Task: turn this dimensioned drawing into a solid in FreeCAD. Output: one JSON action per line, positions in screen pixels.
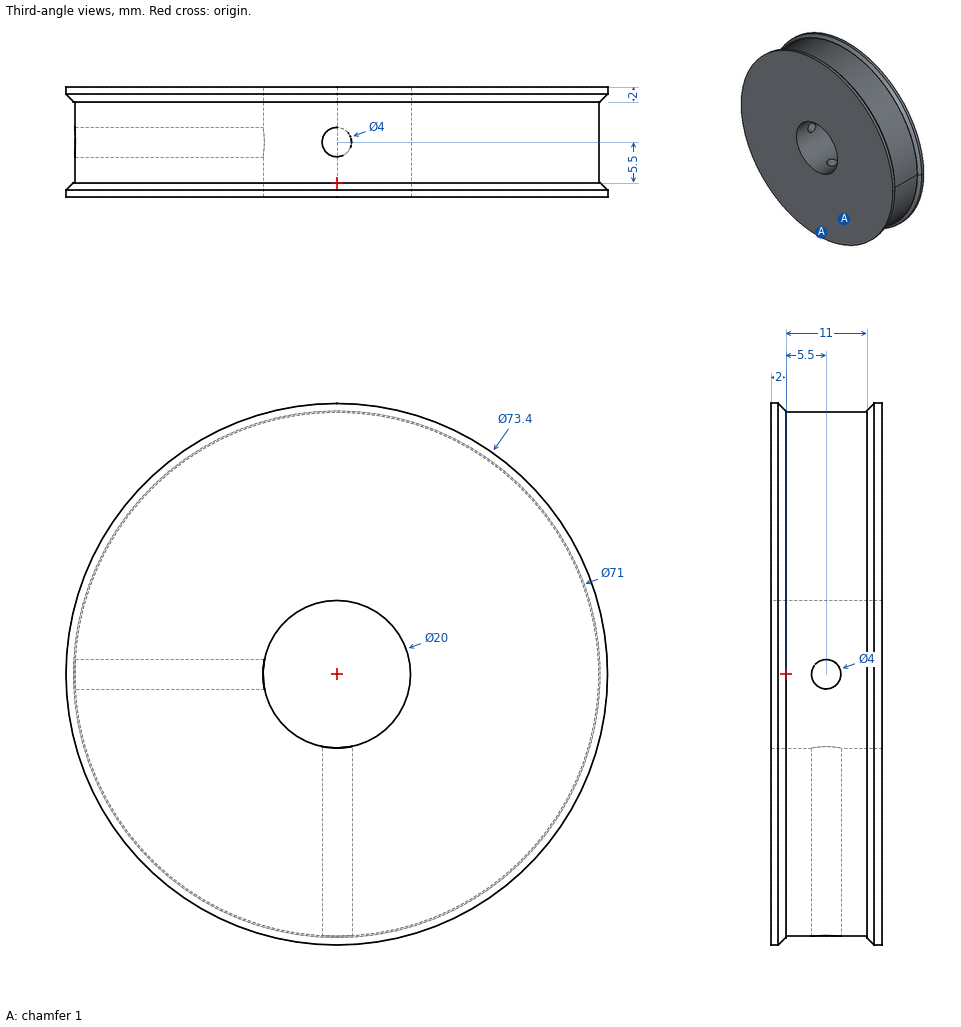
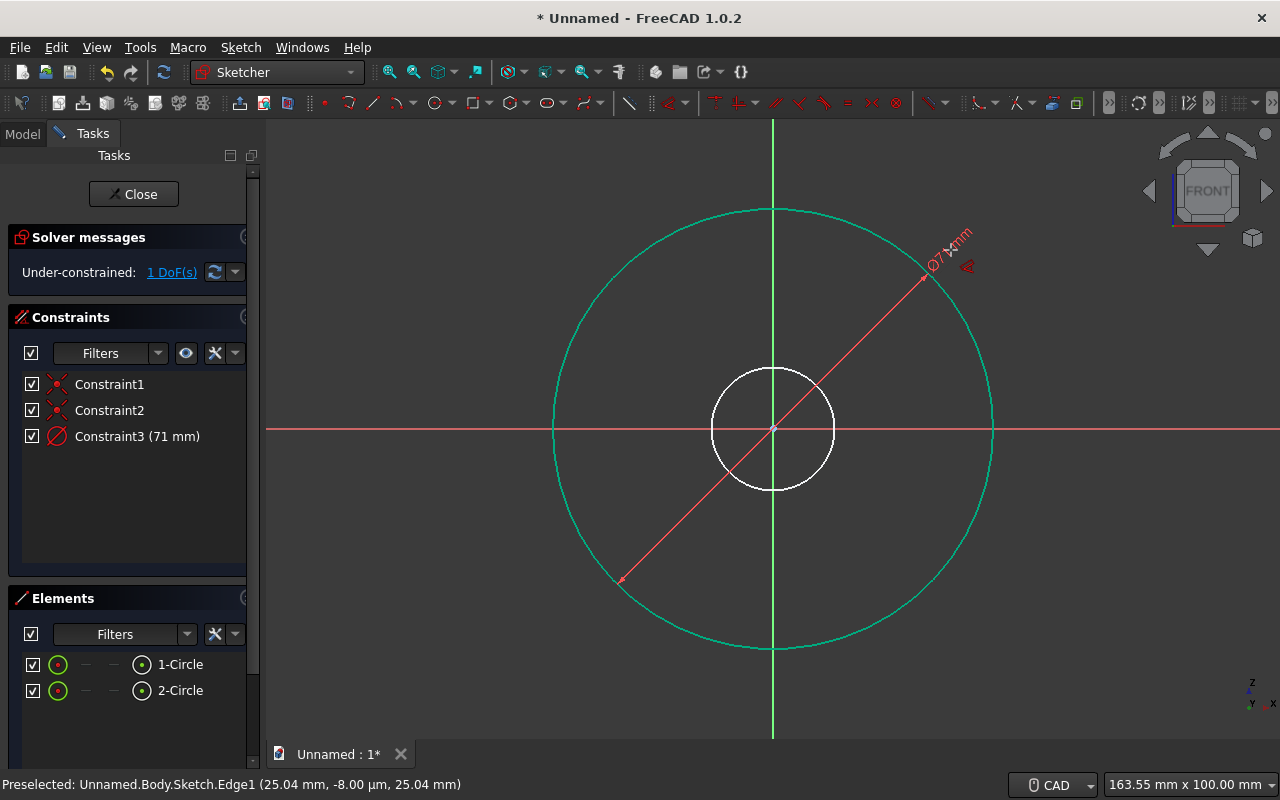
{"action": "left_click", "coordinate": [816, 385]}
{"action": "left_click", "coordinate": [838, 362]}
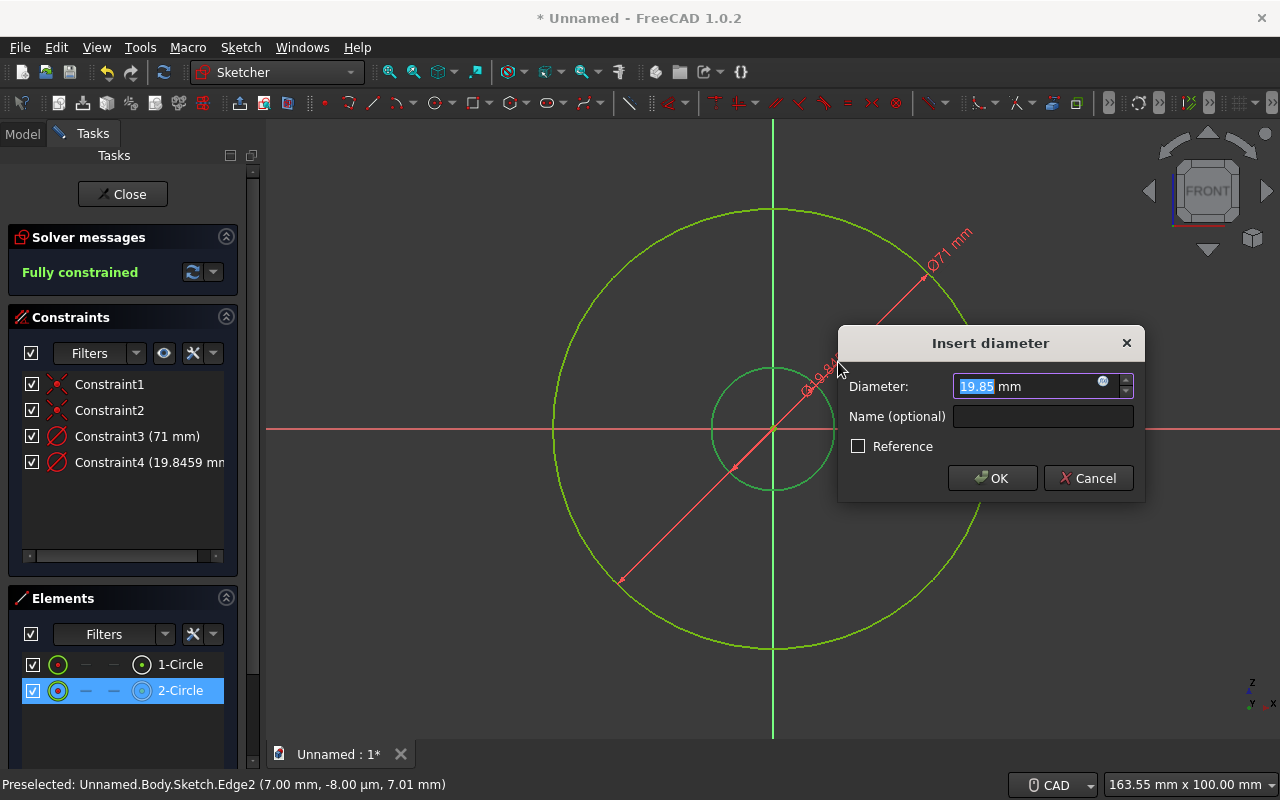
{"action": "type", "text": "20"}
{"action": "key", "text": "Return"}
{"action": "key", "text": "Escape"}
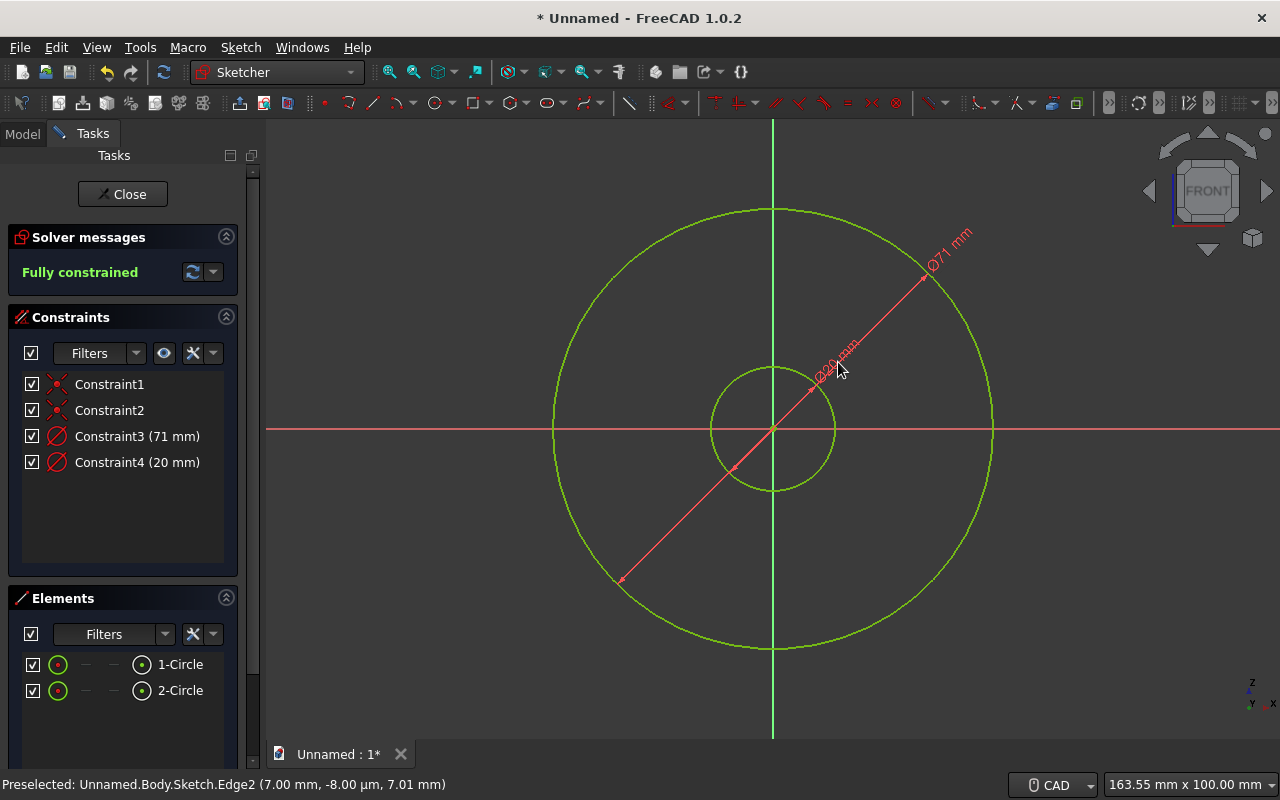
{"action": "left_click", "coordinate": [123, 194]}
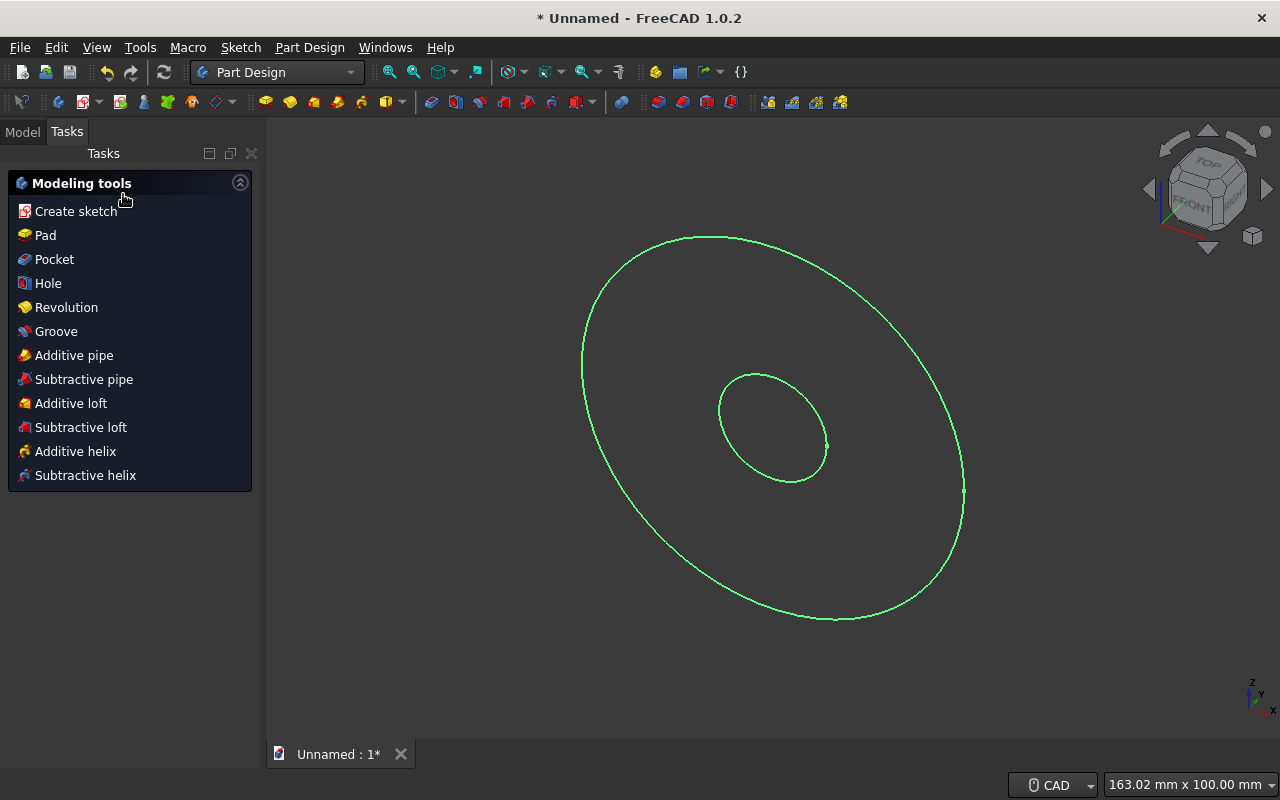
{"action": "left_click", "coordinate": [266, 102]}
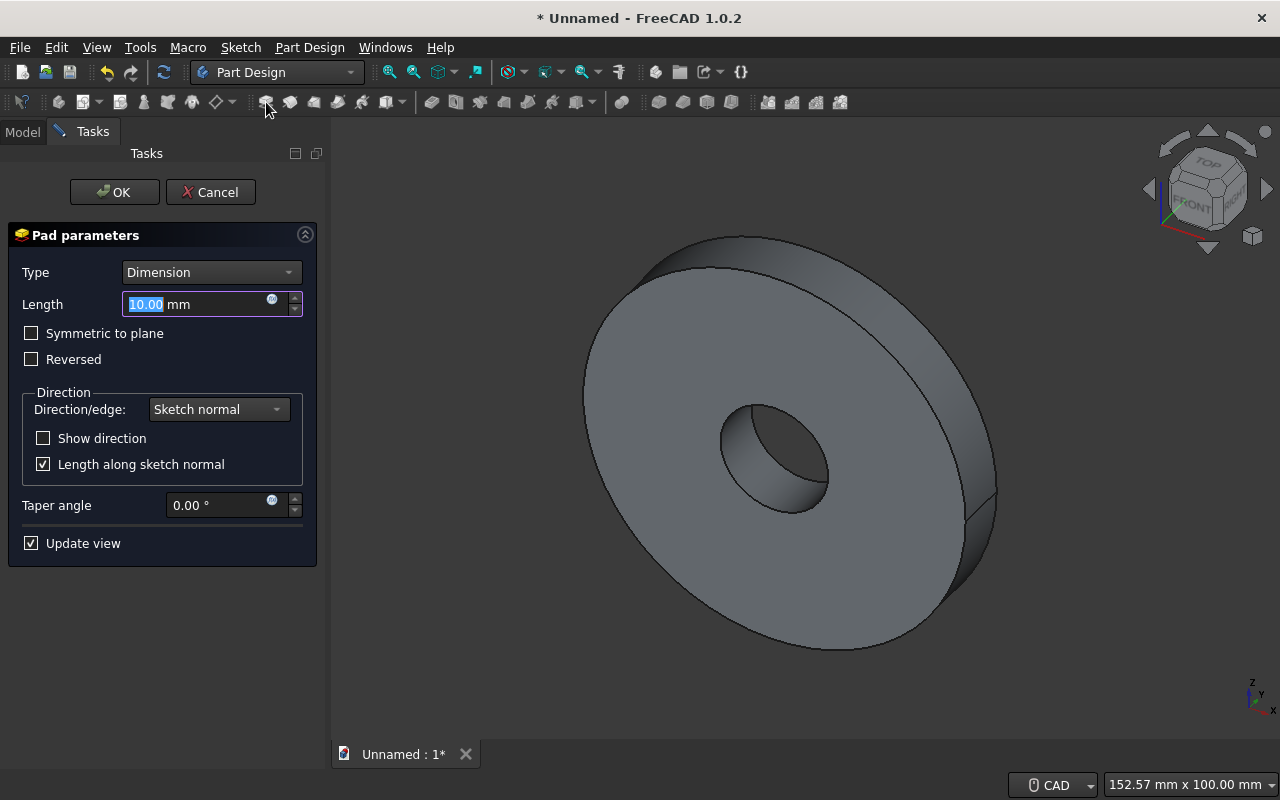
{"action": "type", "text": "11"}
{"action": "key", "text": "Tab"}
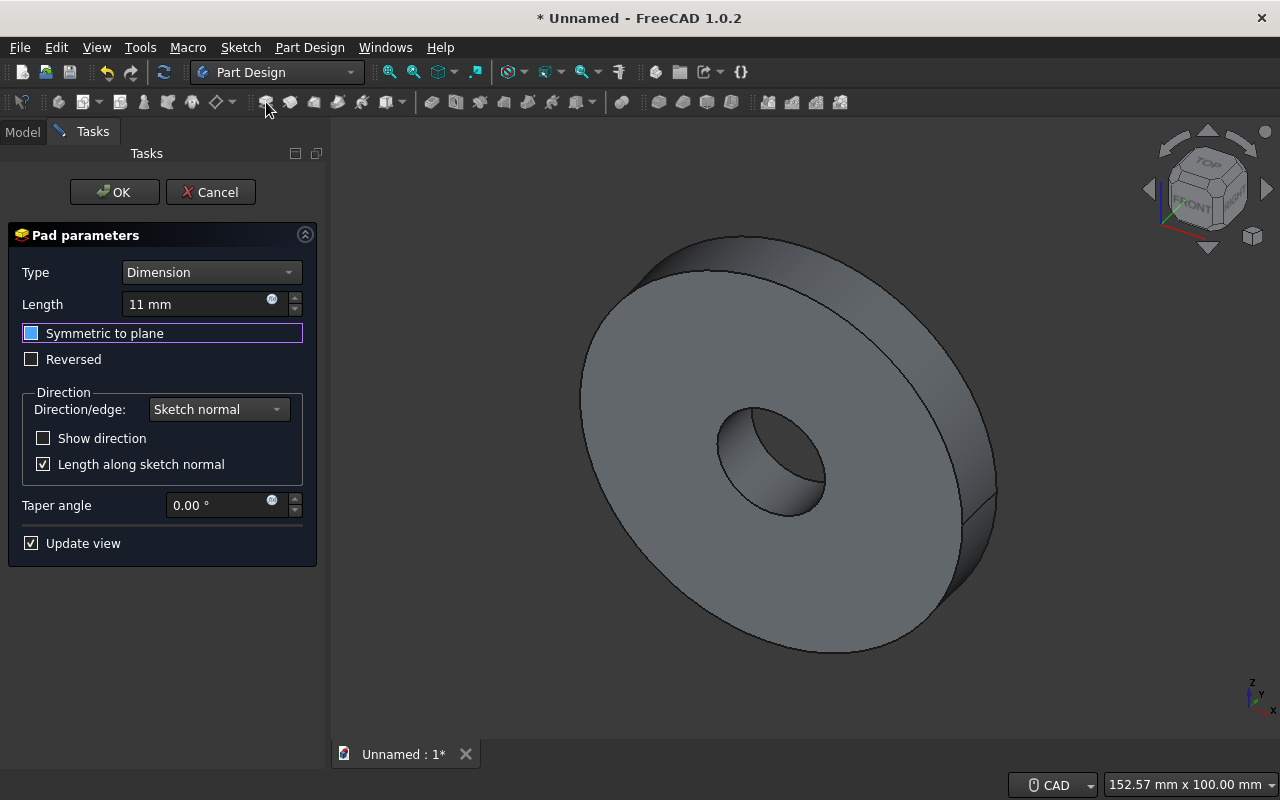
{"action": "left_click", "coordinate": [30, 359]}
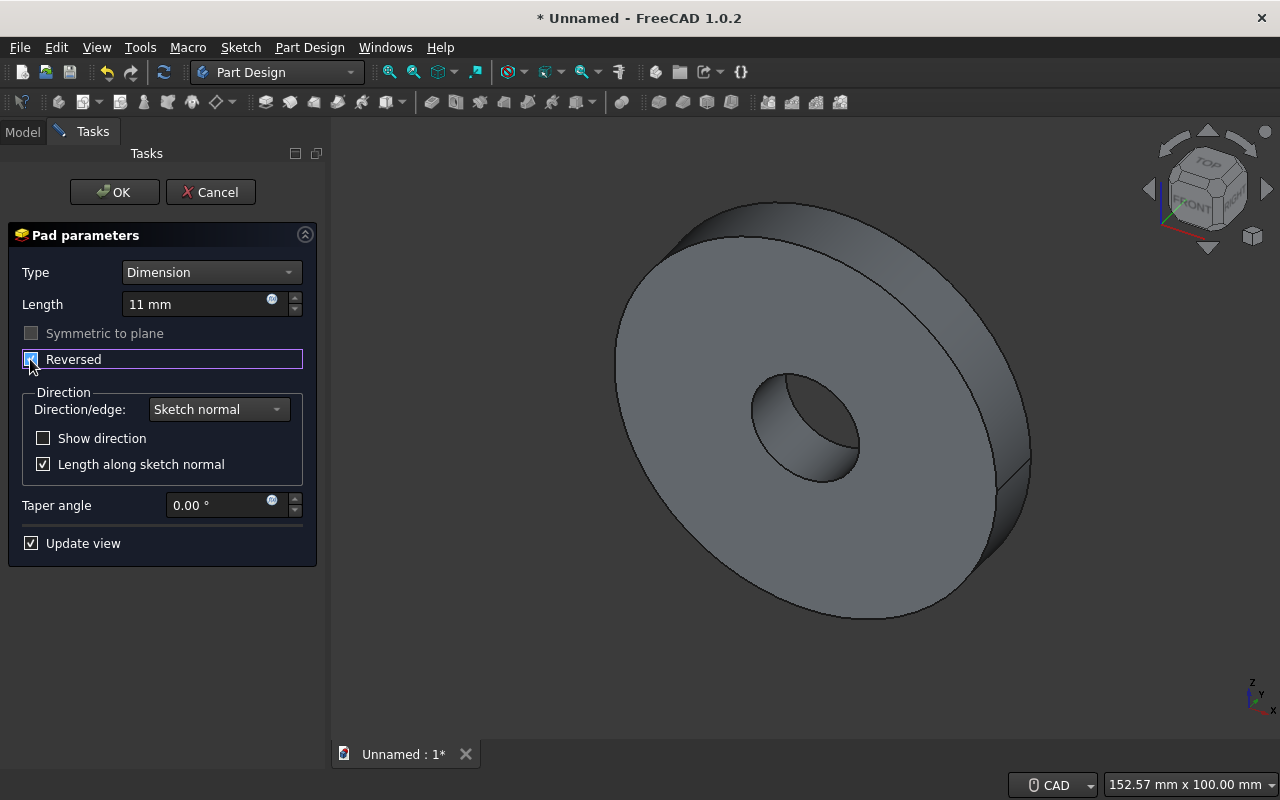
{"action": "left_click", "coordinate": [115, 192]}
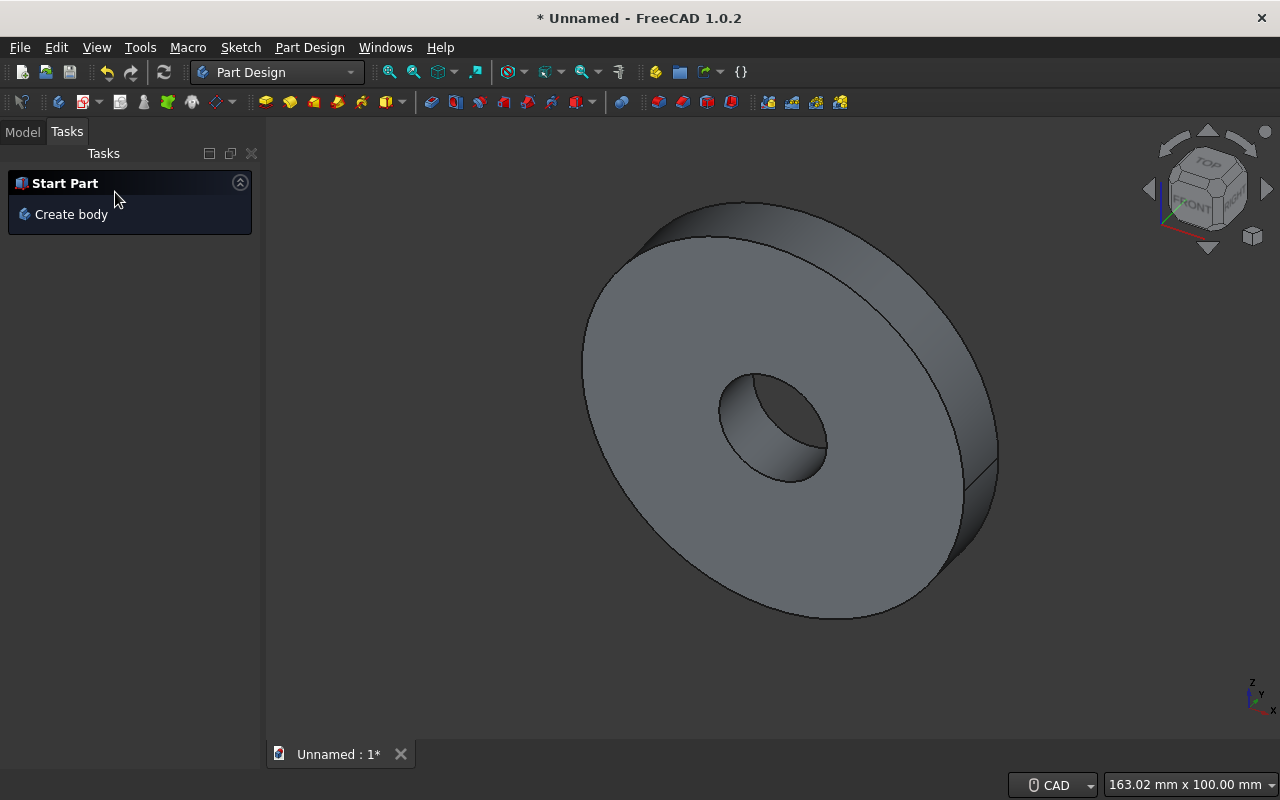
{"action": "key", "text": "4"}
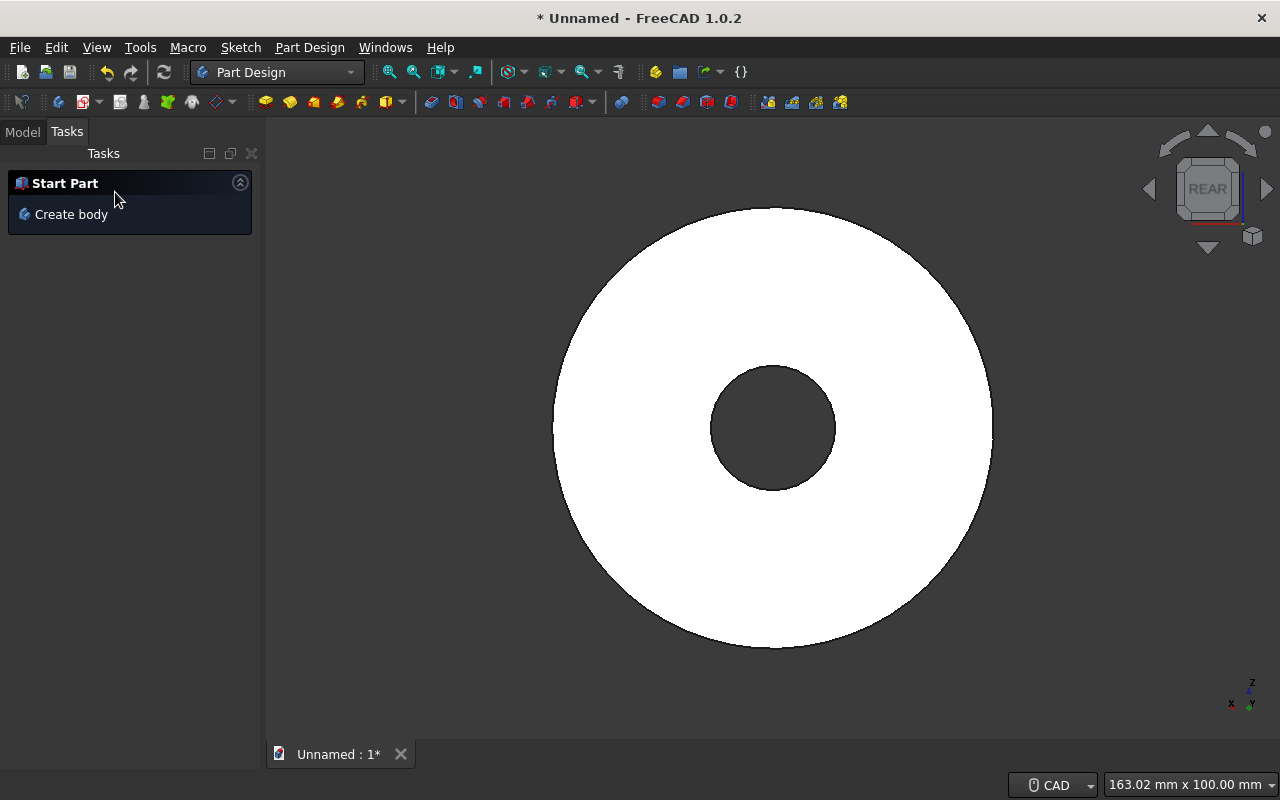
{"action": "left_click", "coordinate": [647, 364]}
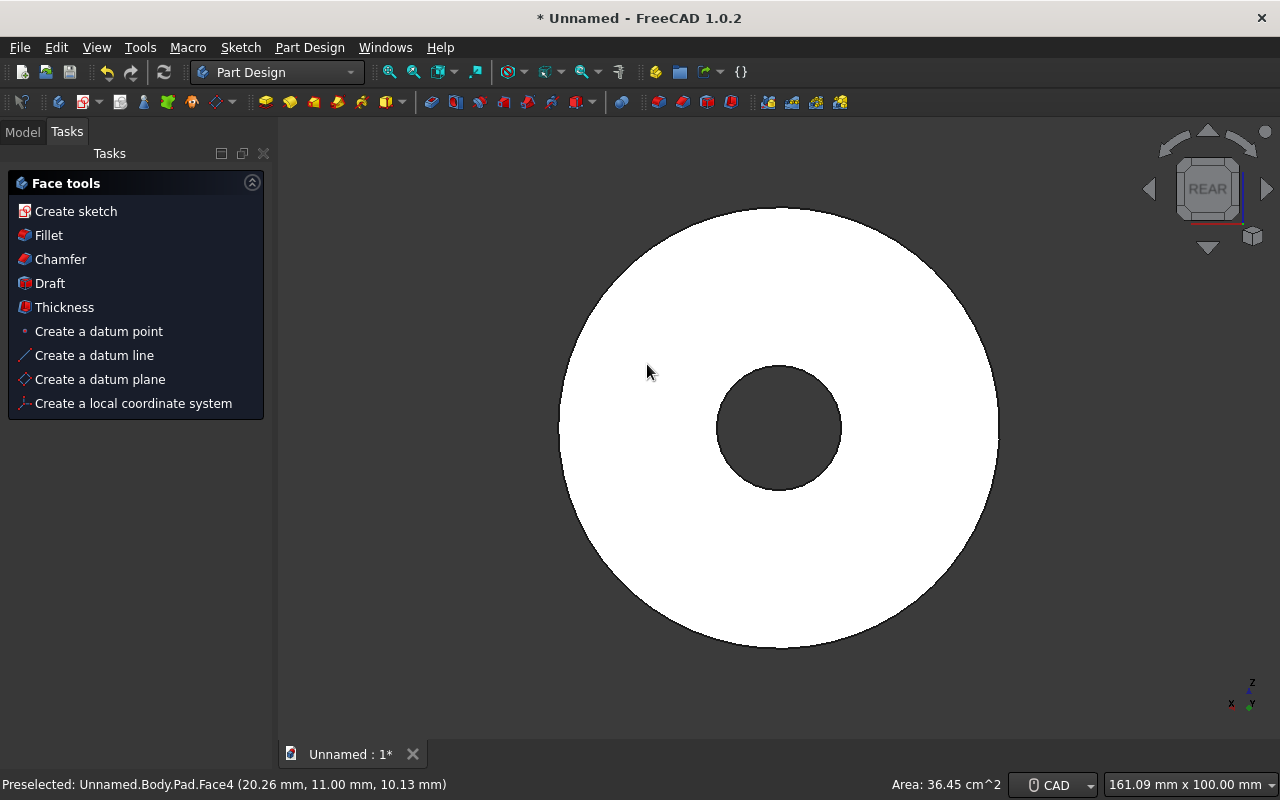
{"action": "left_click", "coordinate": [84, 102]}